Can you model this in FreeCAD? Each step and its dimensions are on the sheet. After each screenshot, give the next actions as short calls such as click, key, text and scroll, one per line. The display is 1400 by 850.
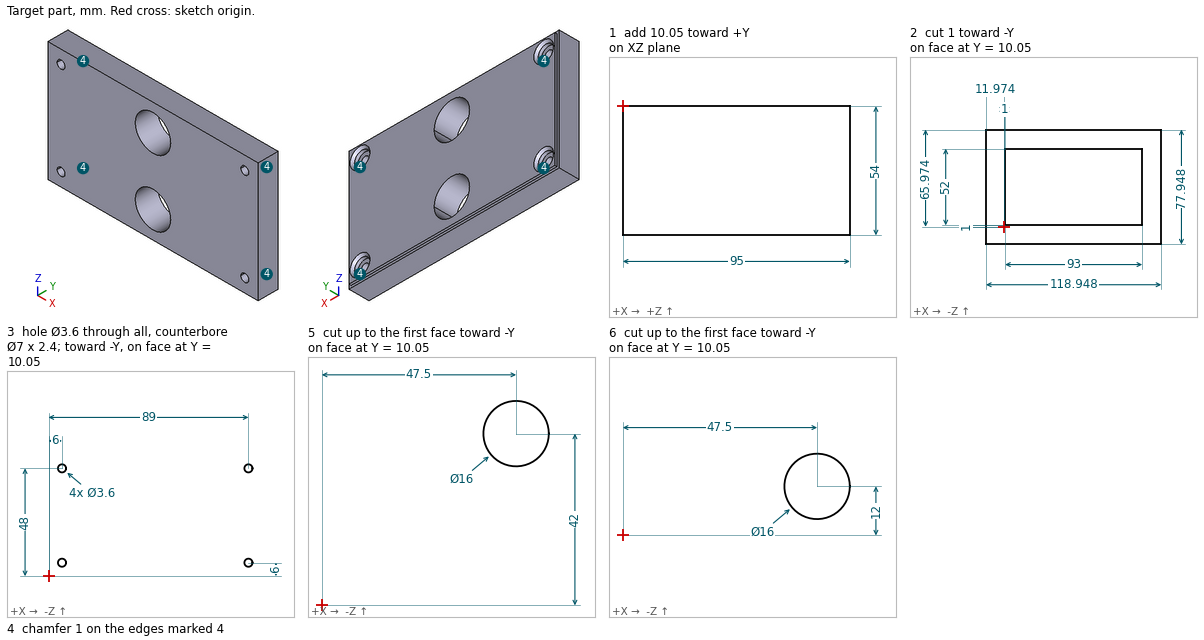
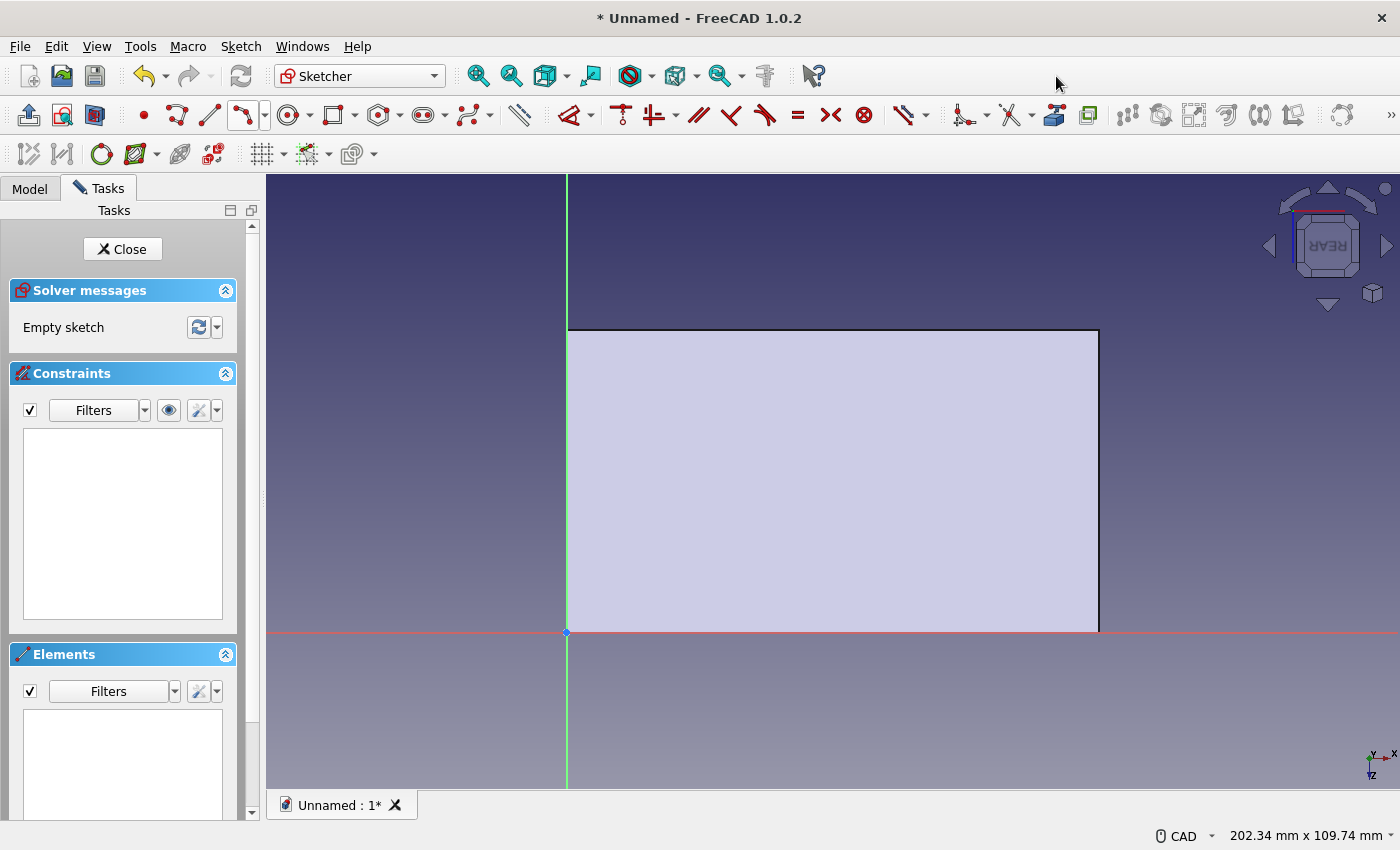
click(332, 116)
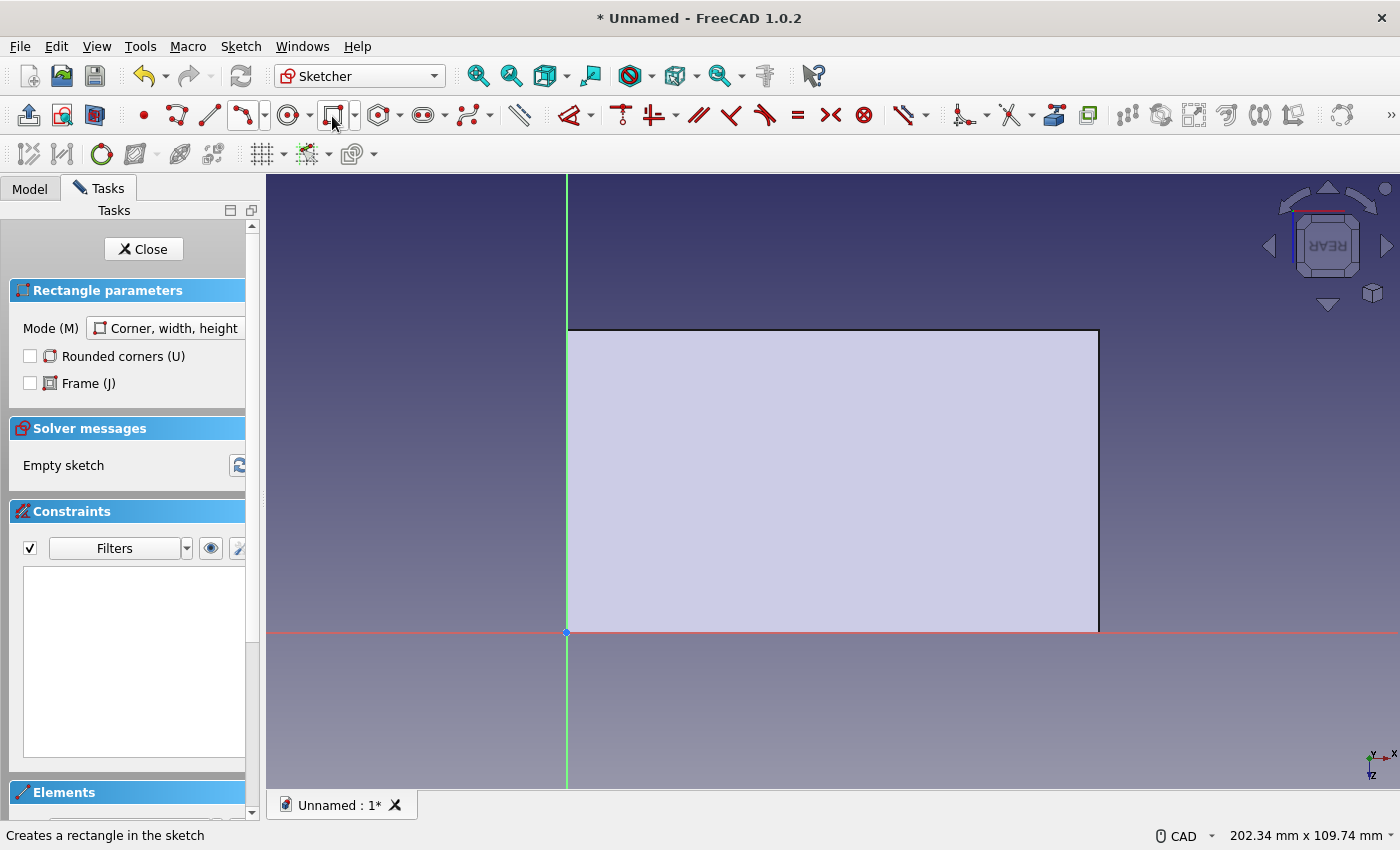
click(500, 263)
move(1166, 700)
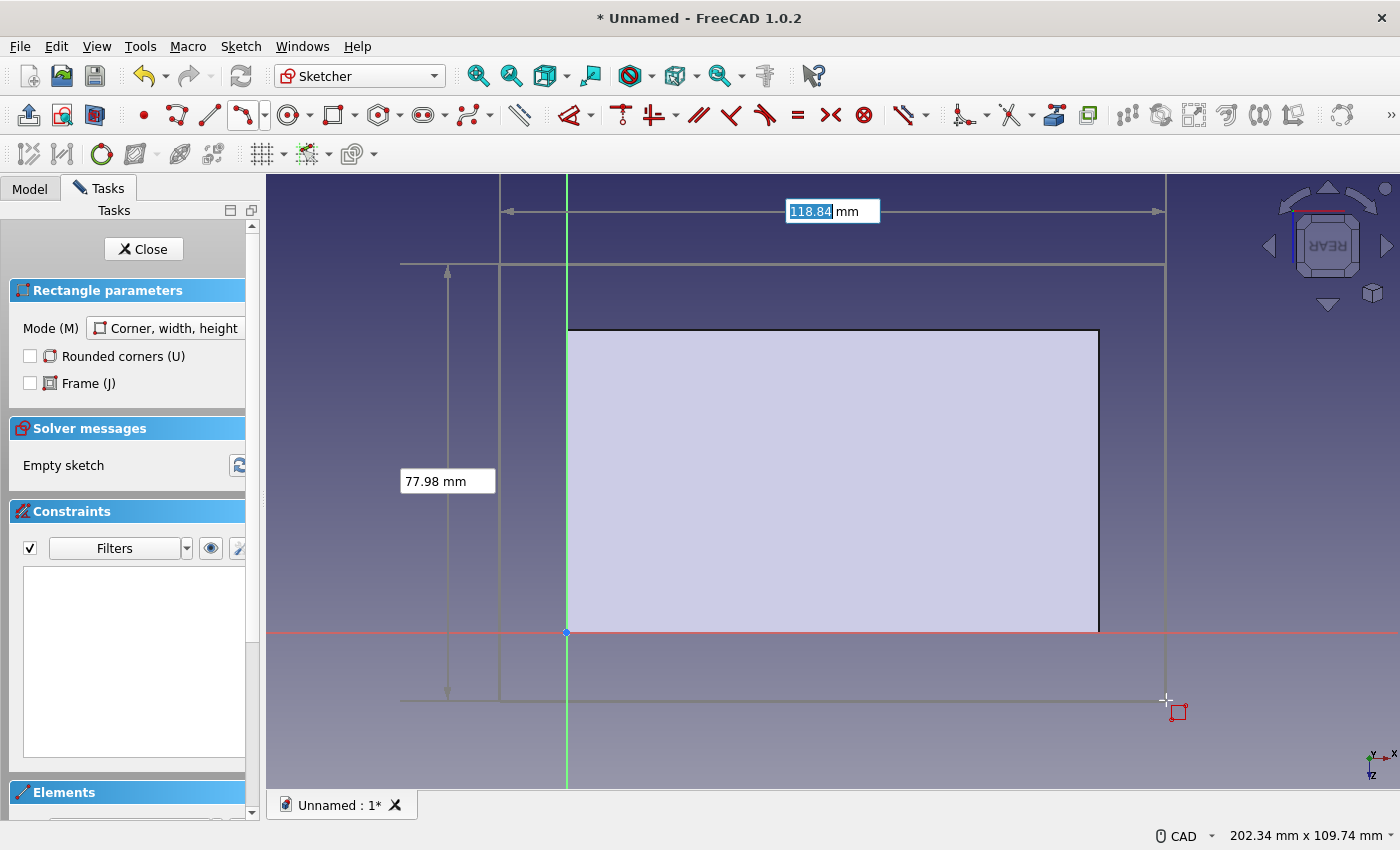
text(118.948)
key(Tab)
text(77.948)
key(Return)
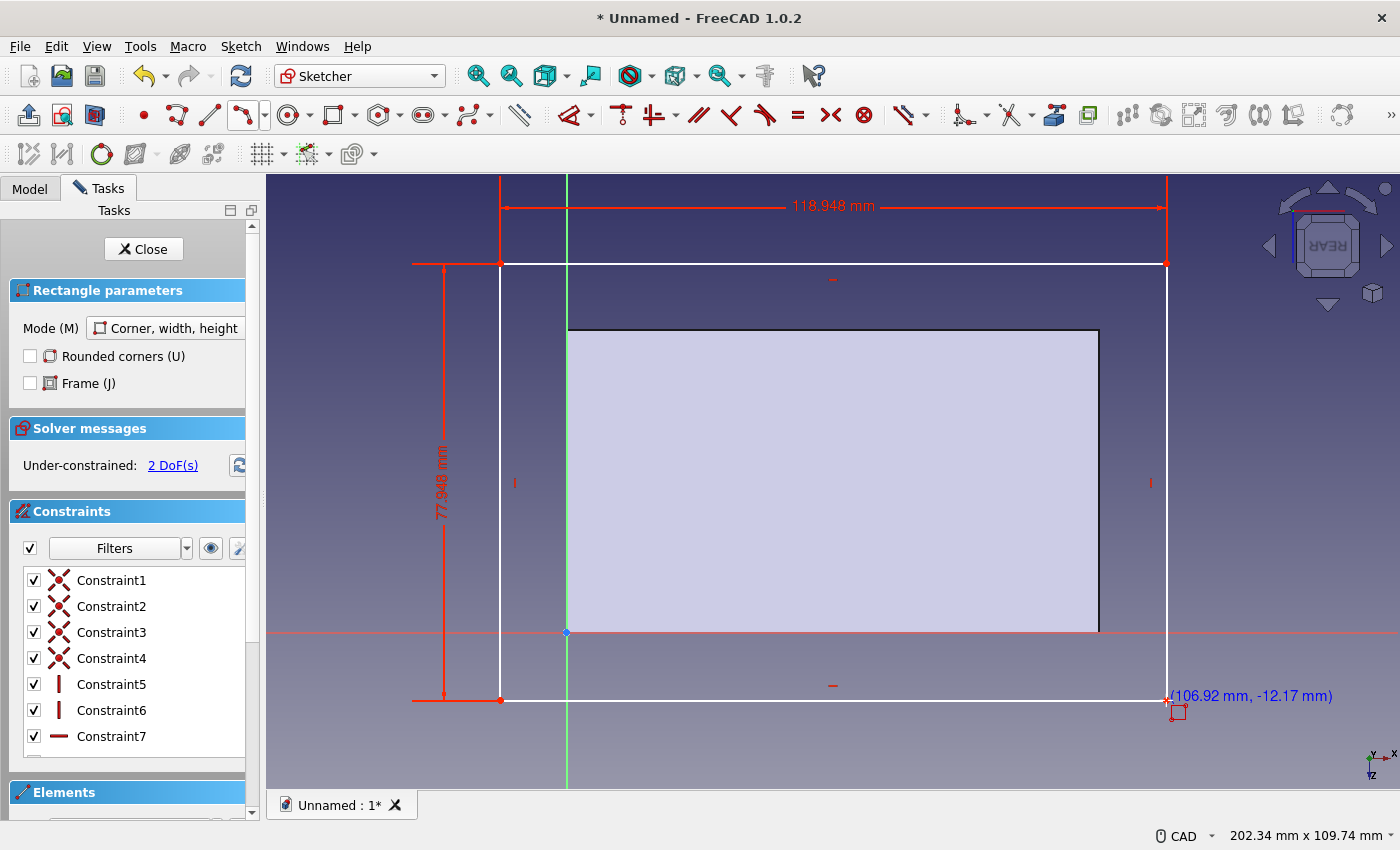
scroll(572, 336, up, 6)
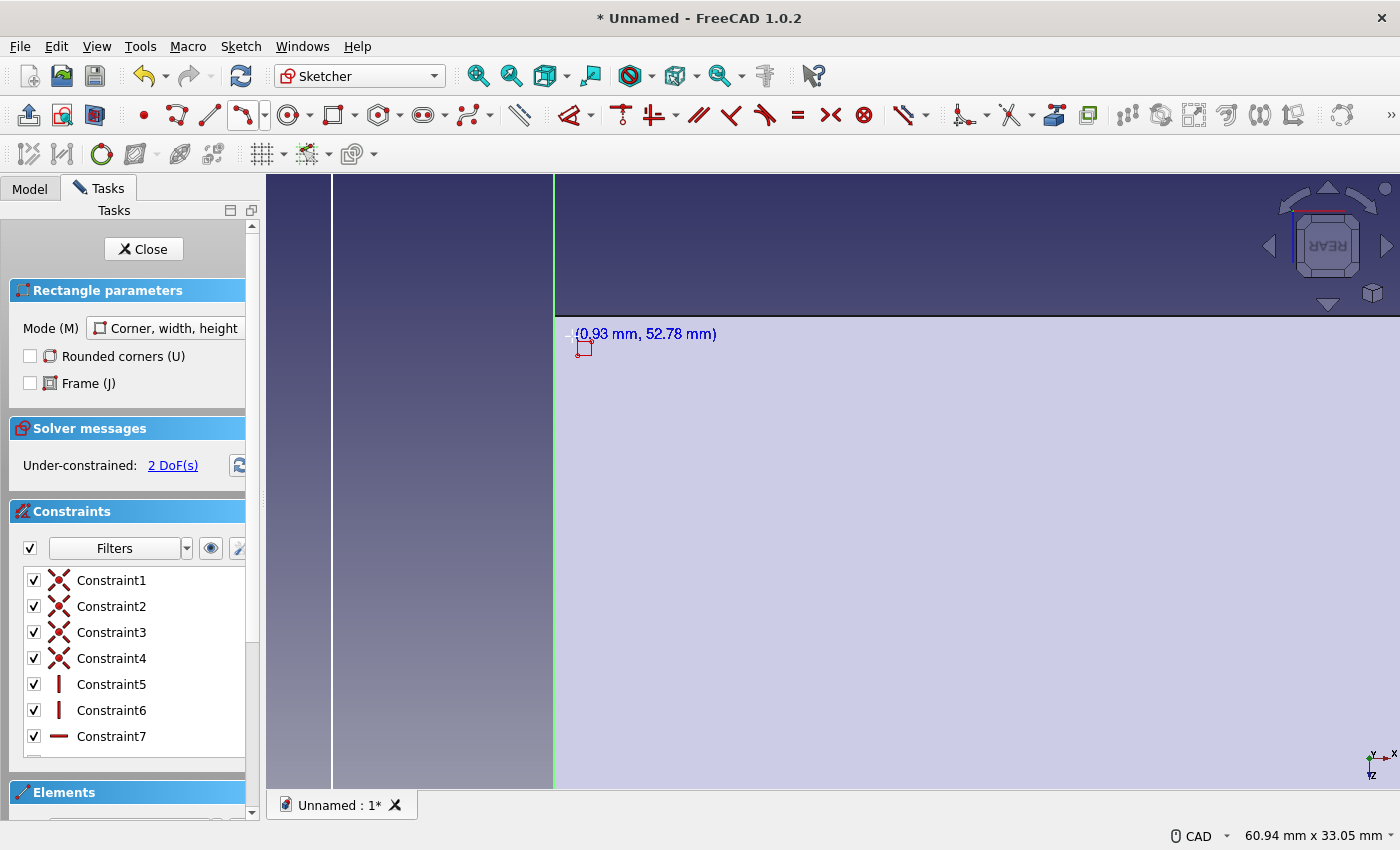
click(573, 335)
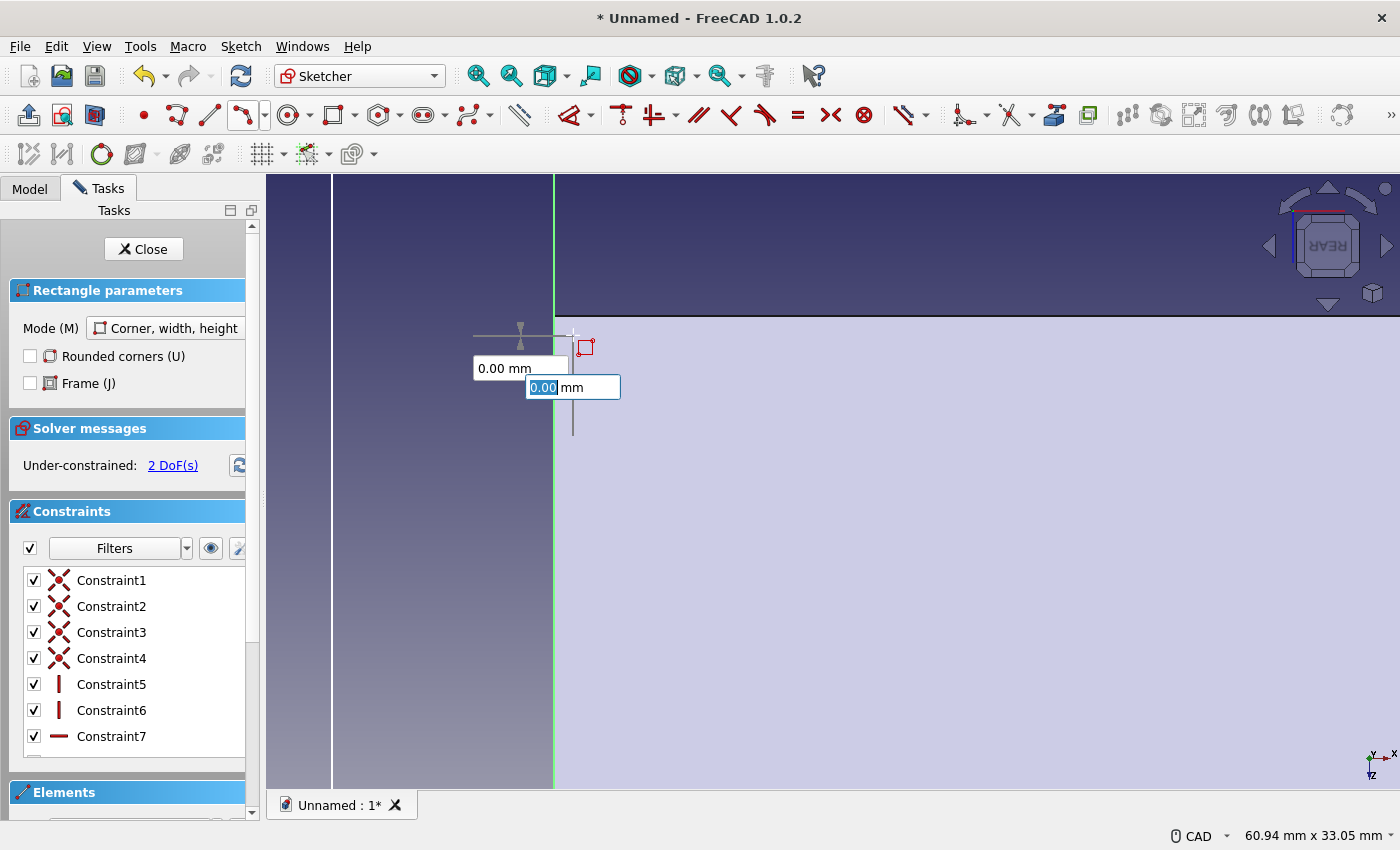
scroll(544, 371, down, 7)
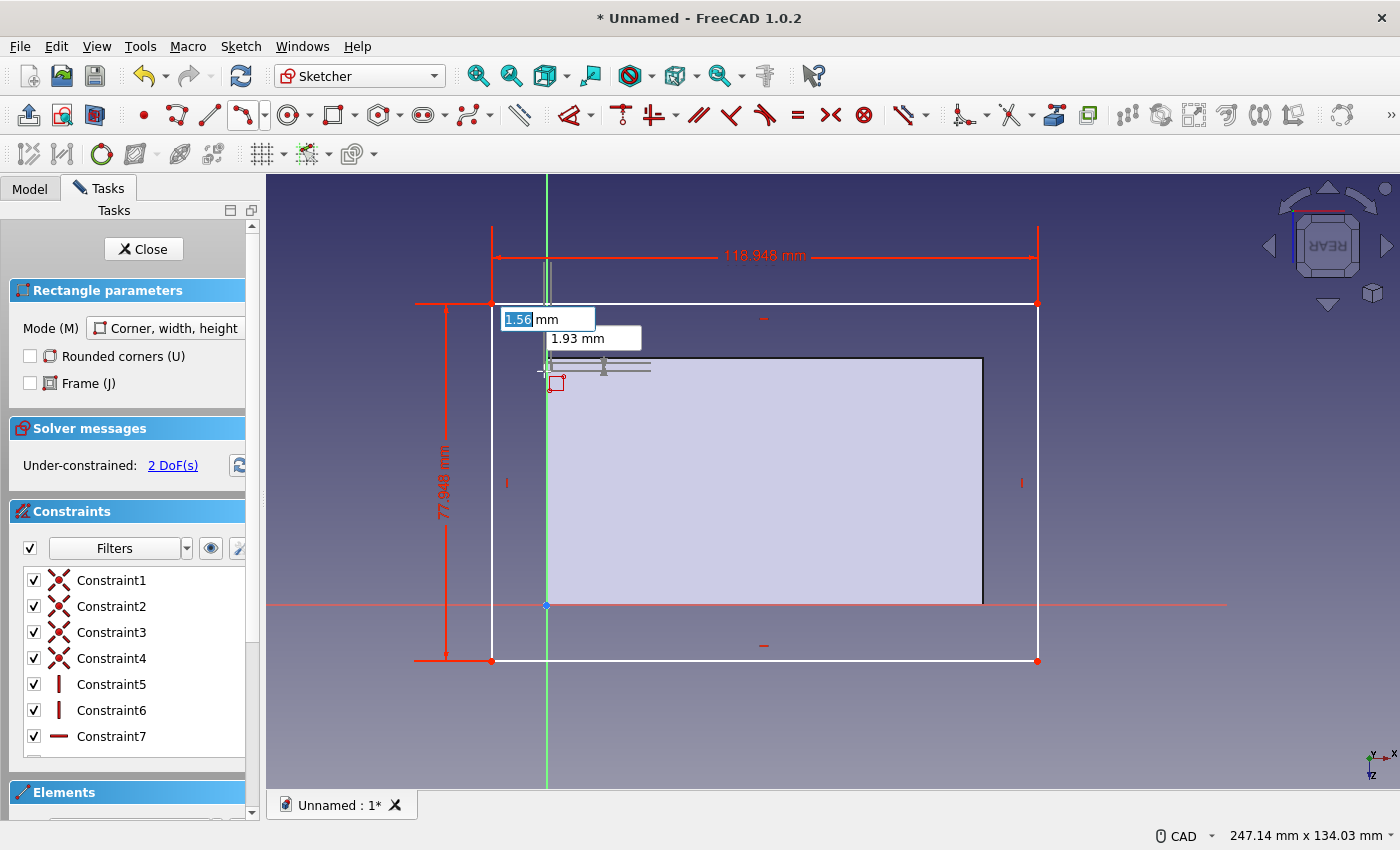
scroll(978, 601, up, 7)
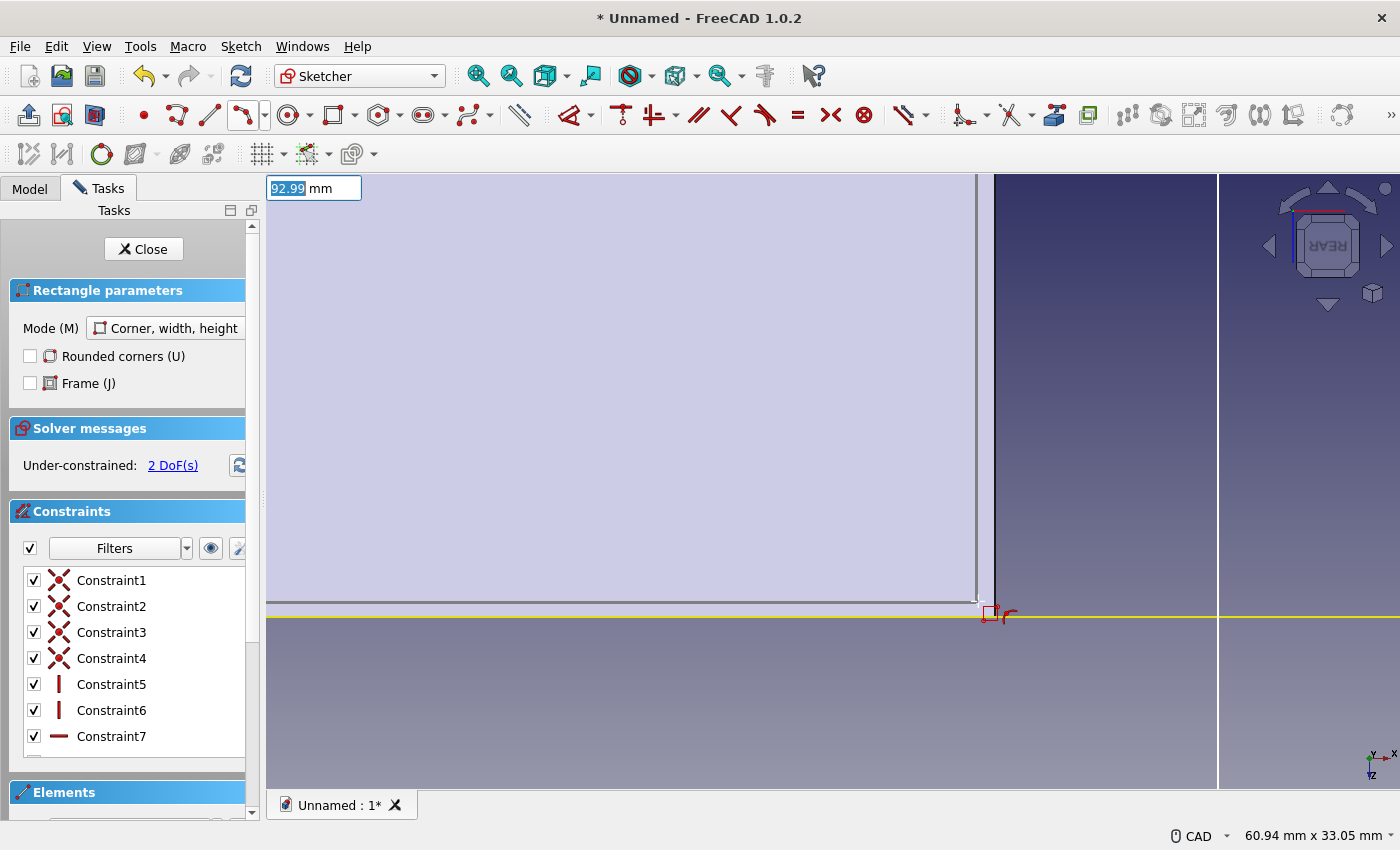
click(976, 598)
key(Escape)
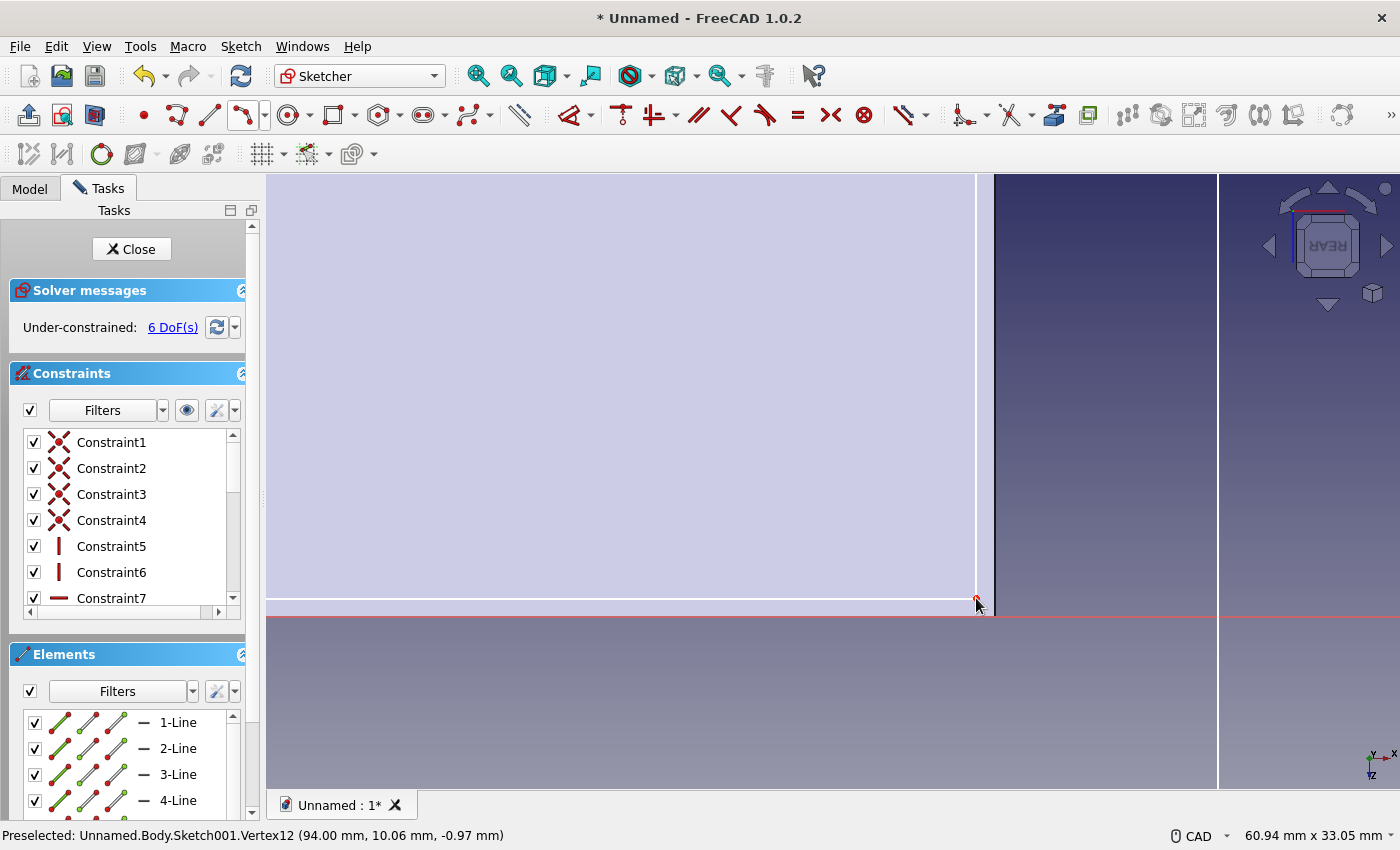
click(568, 116)